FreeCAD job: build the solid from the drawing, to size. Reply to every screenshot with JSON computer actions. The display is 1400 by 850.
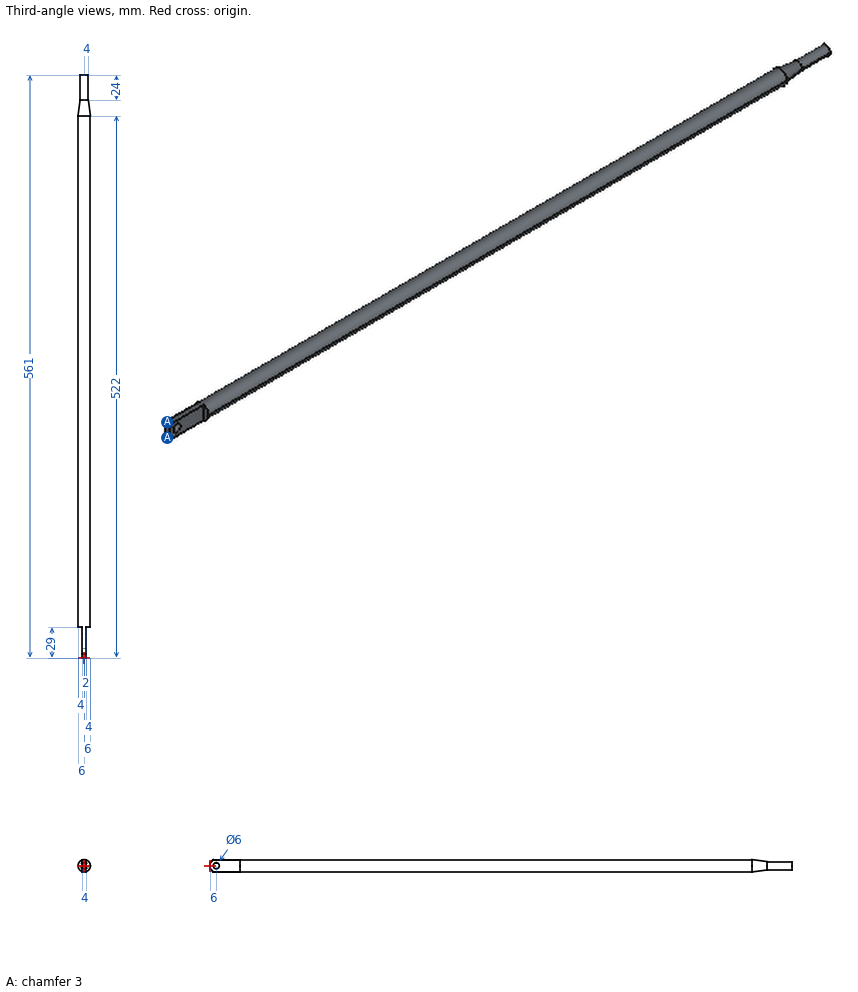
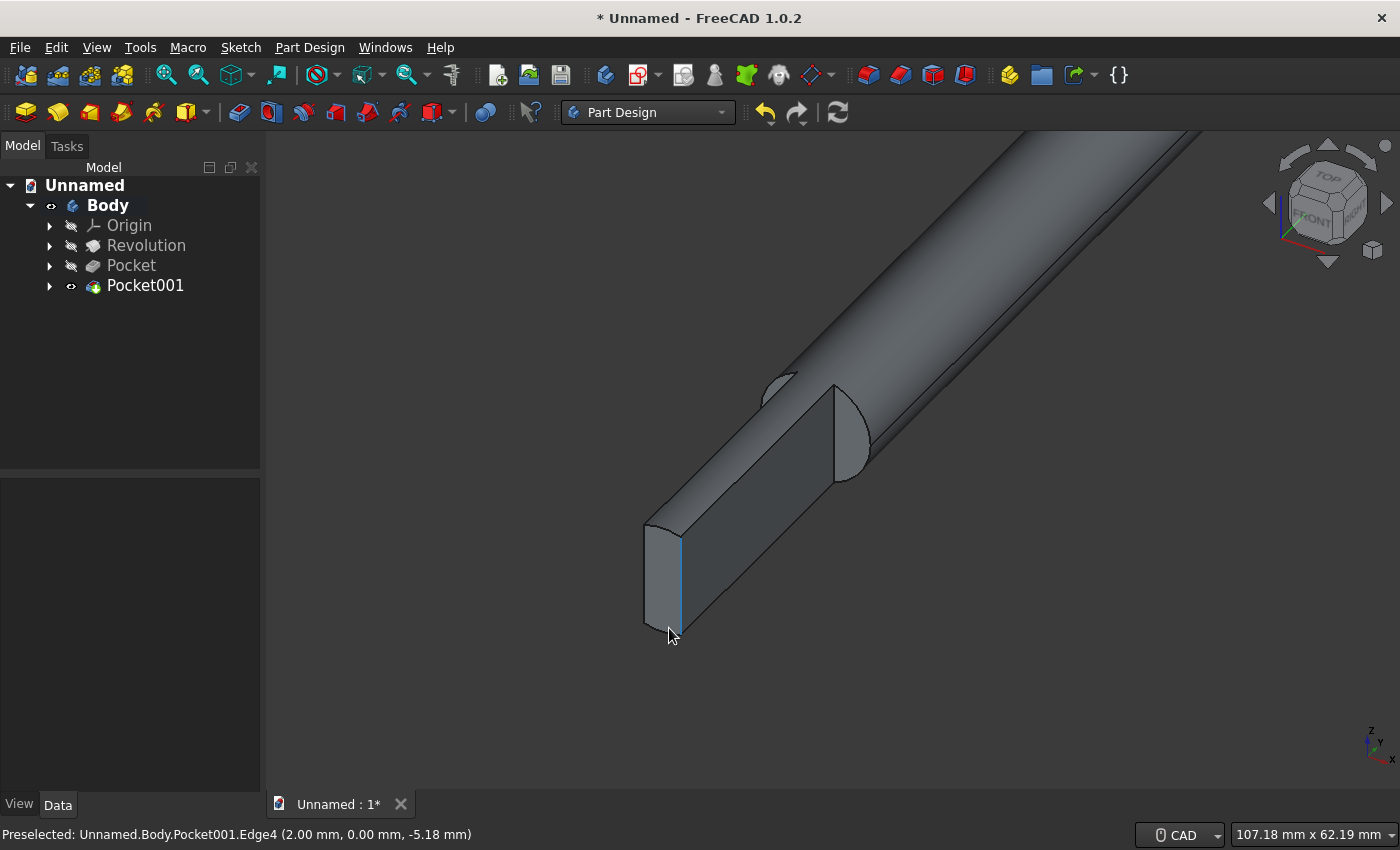
{"action": "left_click", "coordinate": [662, 527]}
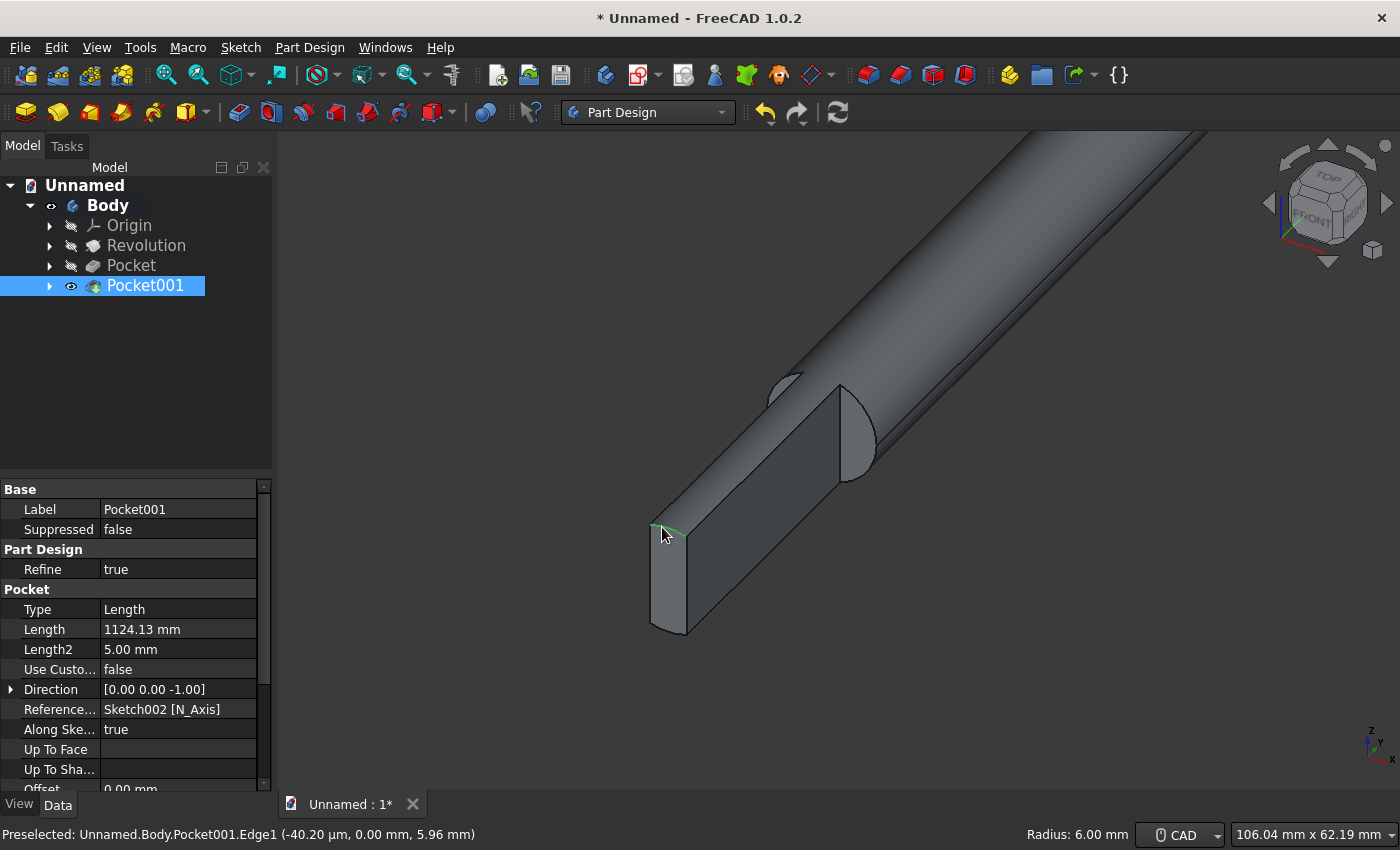
{"action": "left_click", "coordinate": [168, 76]}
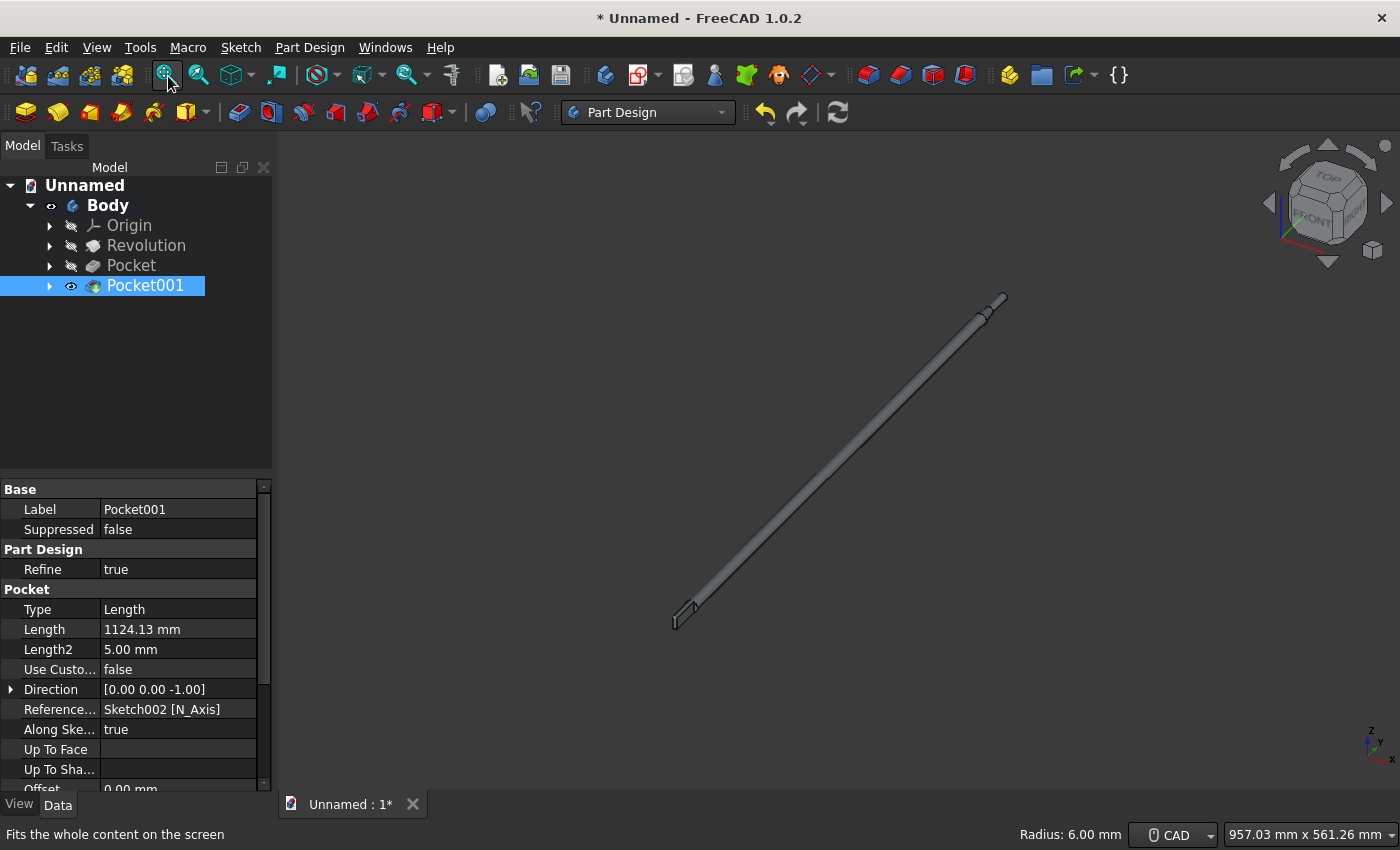
{"action": "key", "text": "0"}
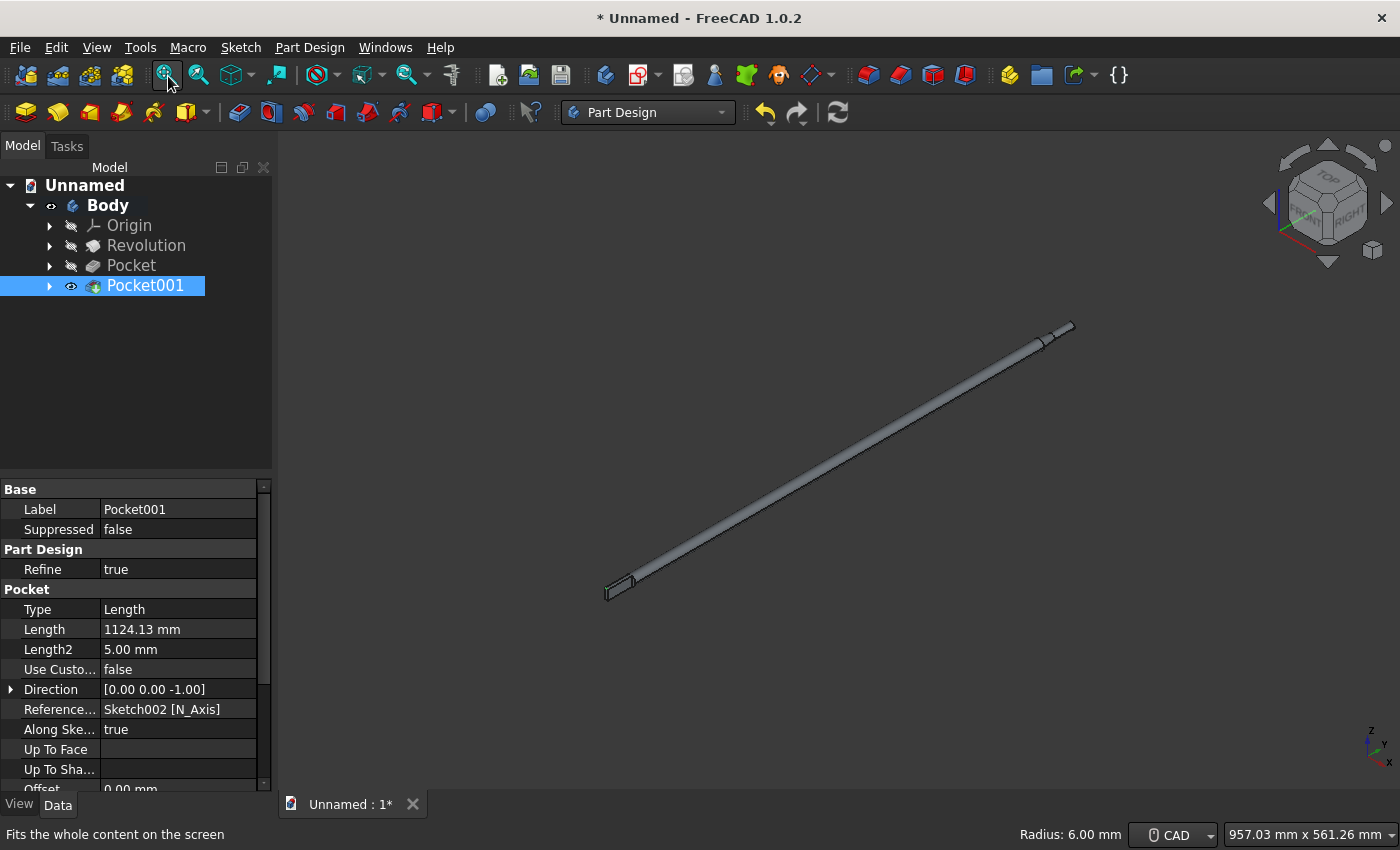
{"action": "left_click", "coordinate": [168, 76]}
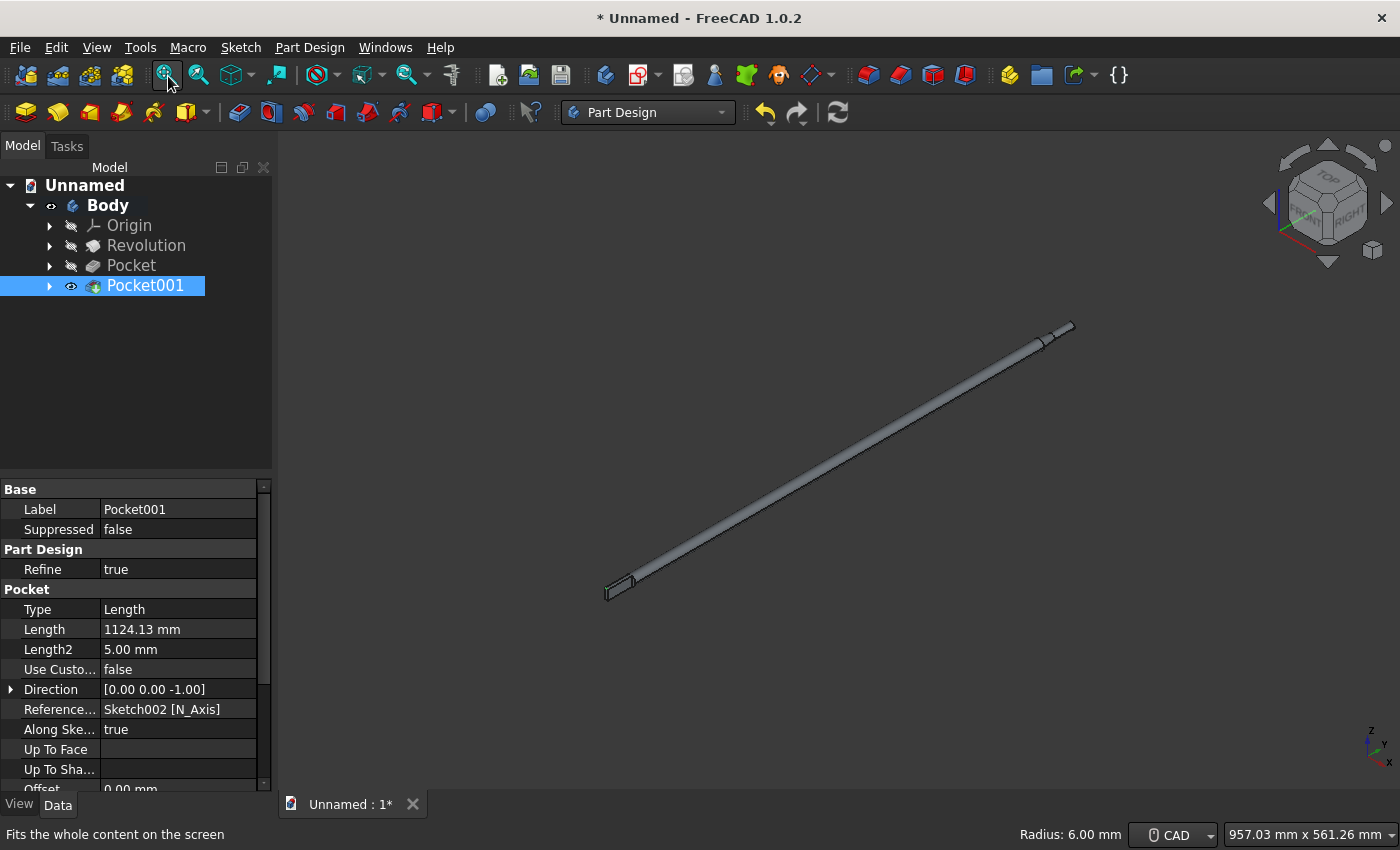
{"action": "scroll", "coordinate": [606, 599], "scroll_direction": "up", "scroll_amount": 11}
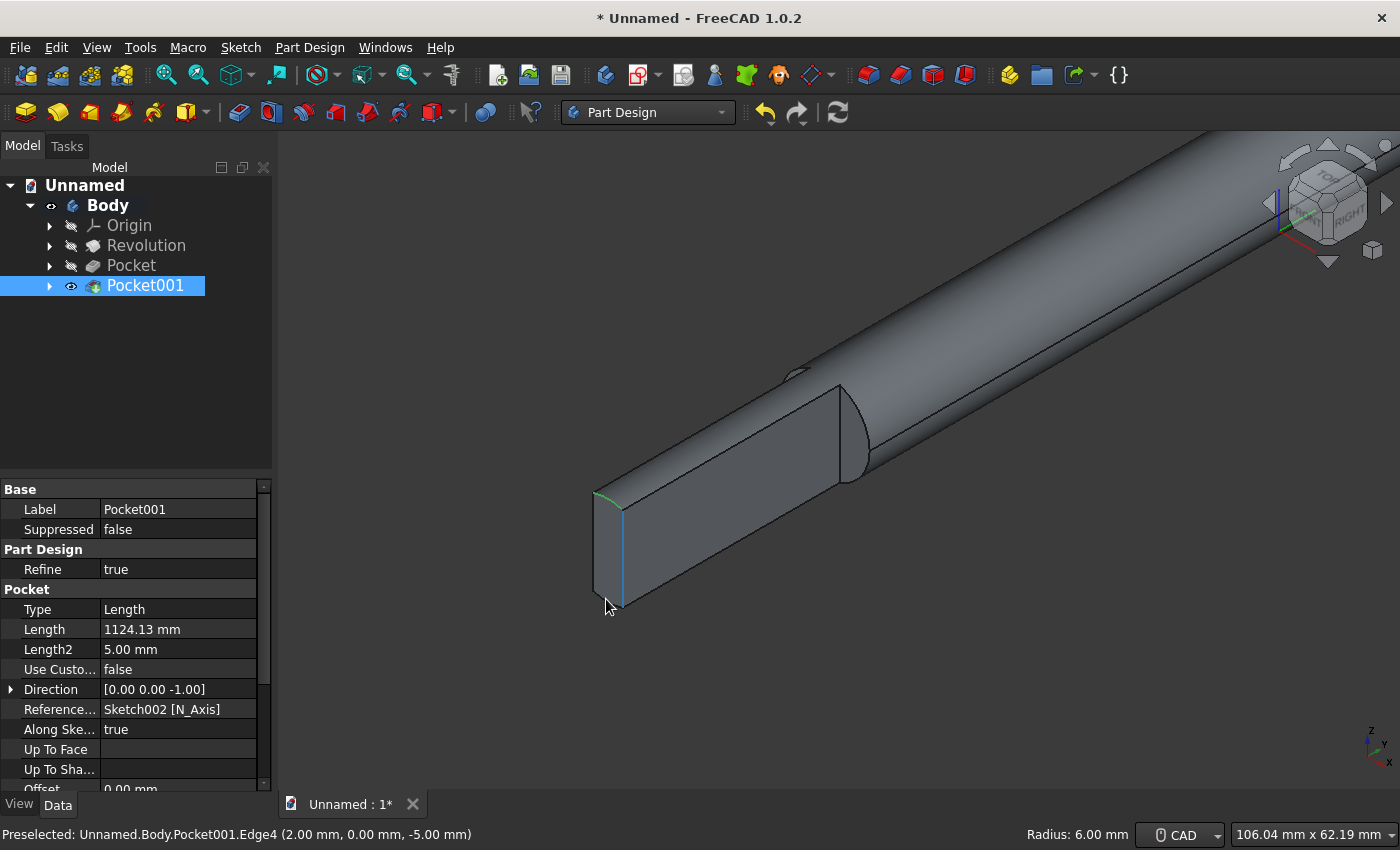
{"action": "left_click", "coordinate": [168, 76]}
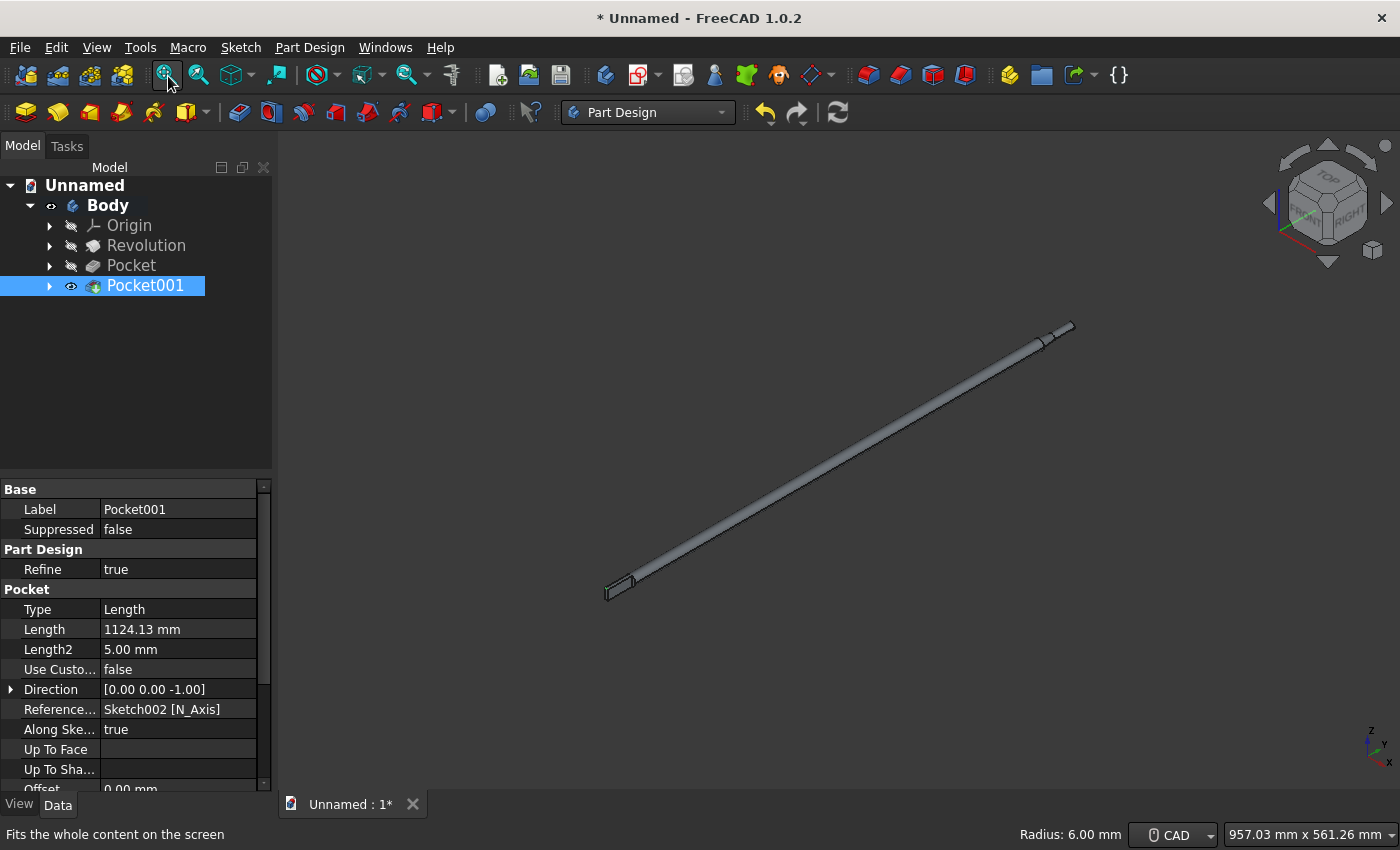
{"action": "key", "text": "2"}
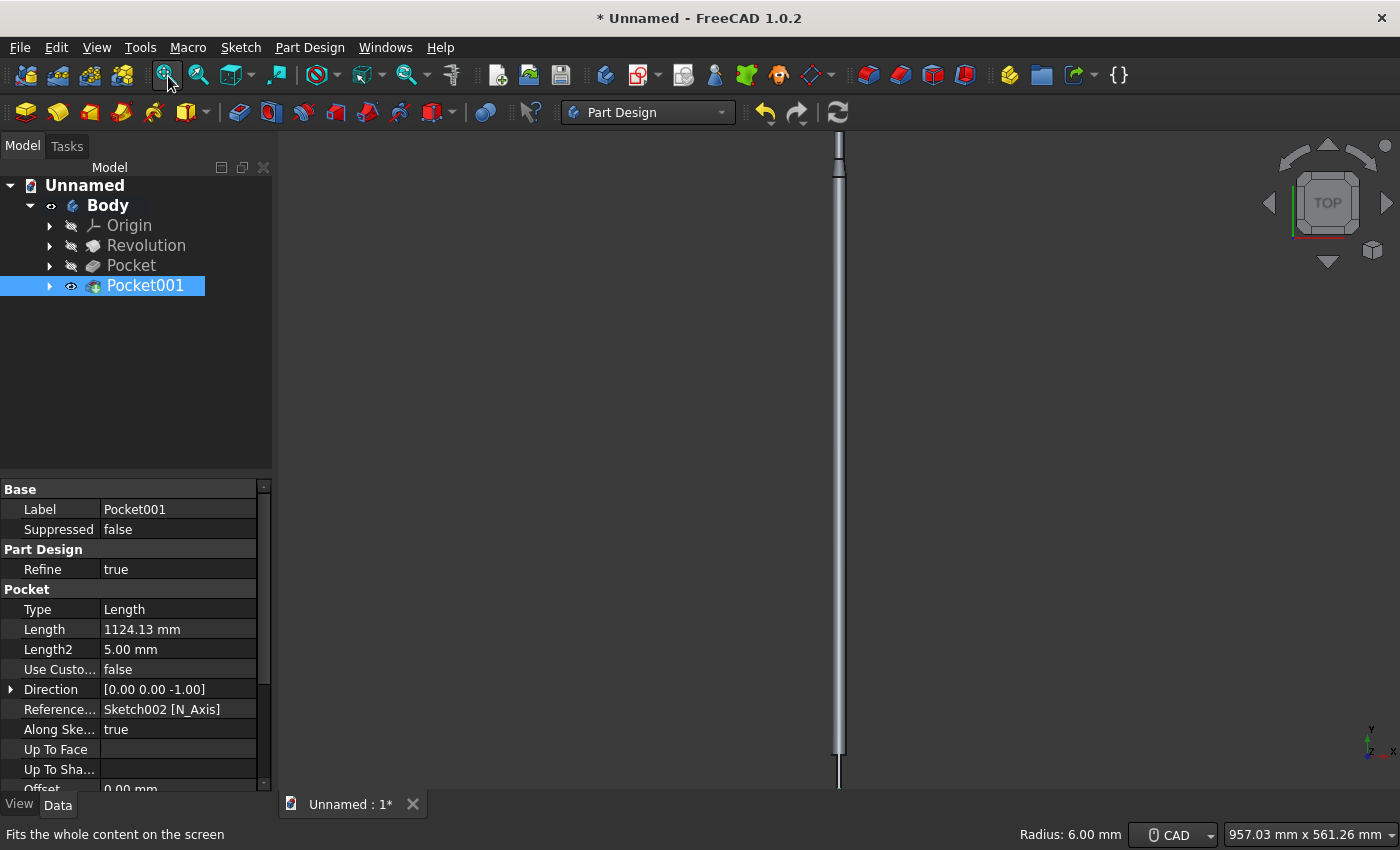
{"action": "left_click", "coordinate": [168, 76]}